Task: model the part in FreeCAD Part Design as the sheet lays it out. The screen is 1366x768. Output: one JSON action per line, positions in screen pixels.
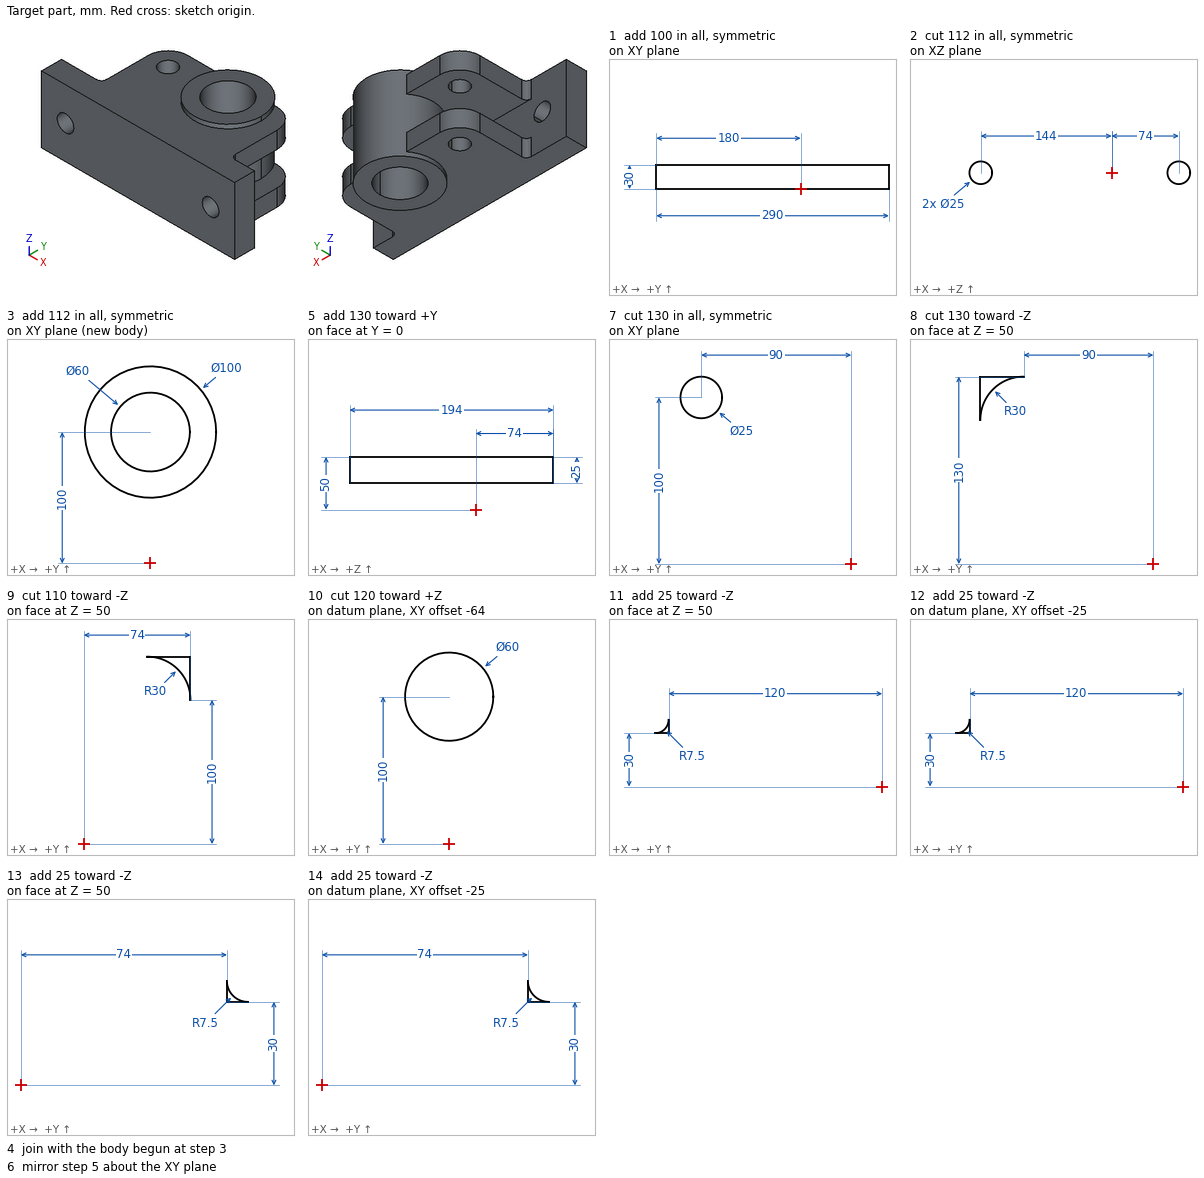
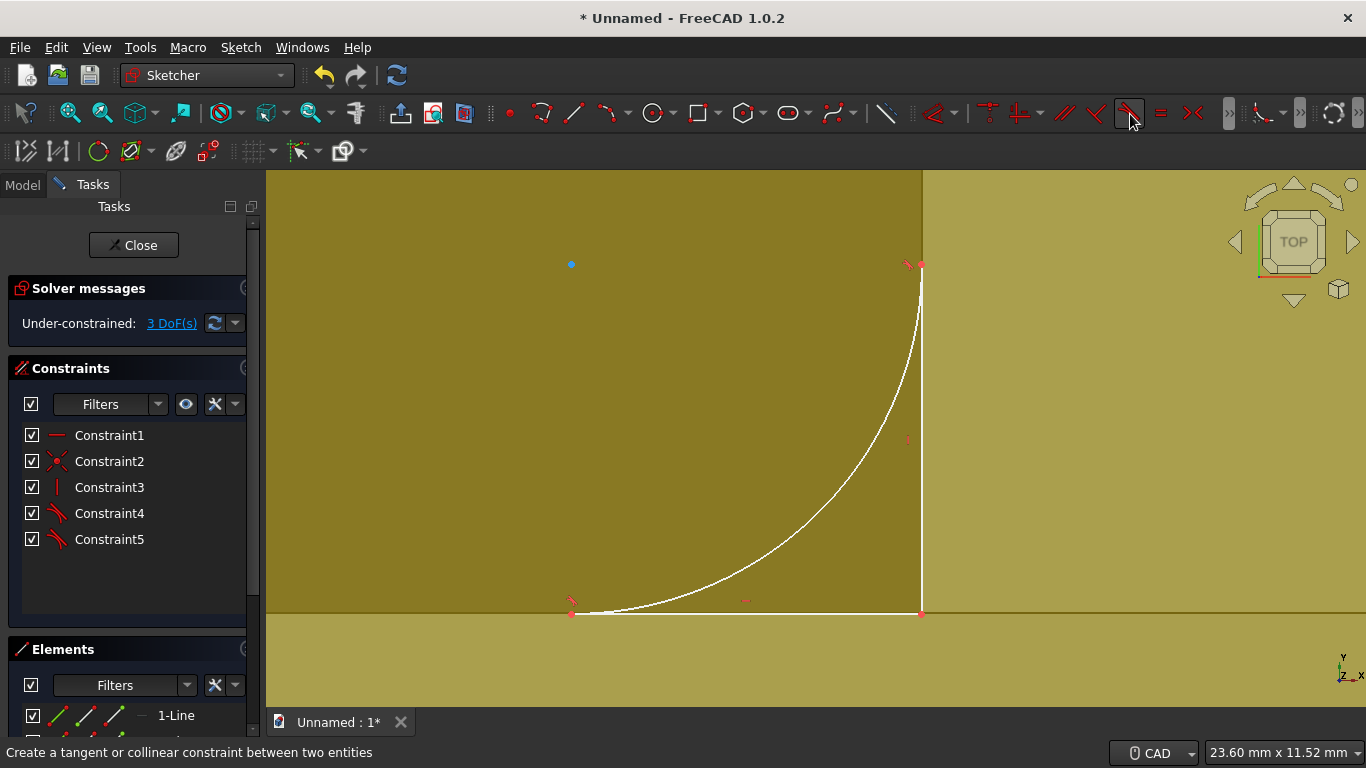
{"action": "left_click", "coordinate": [934, 114]}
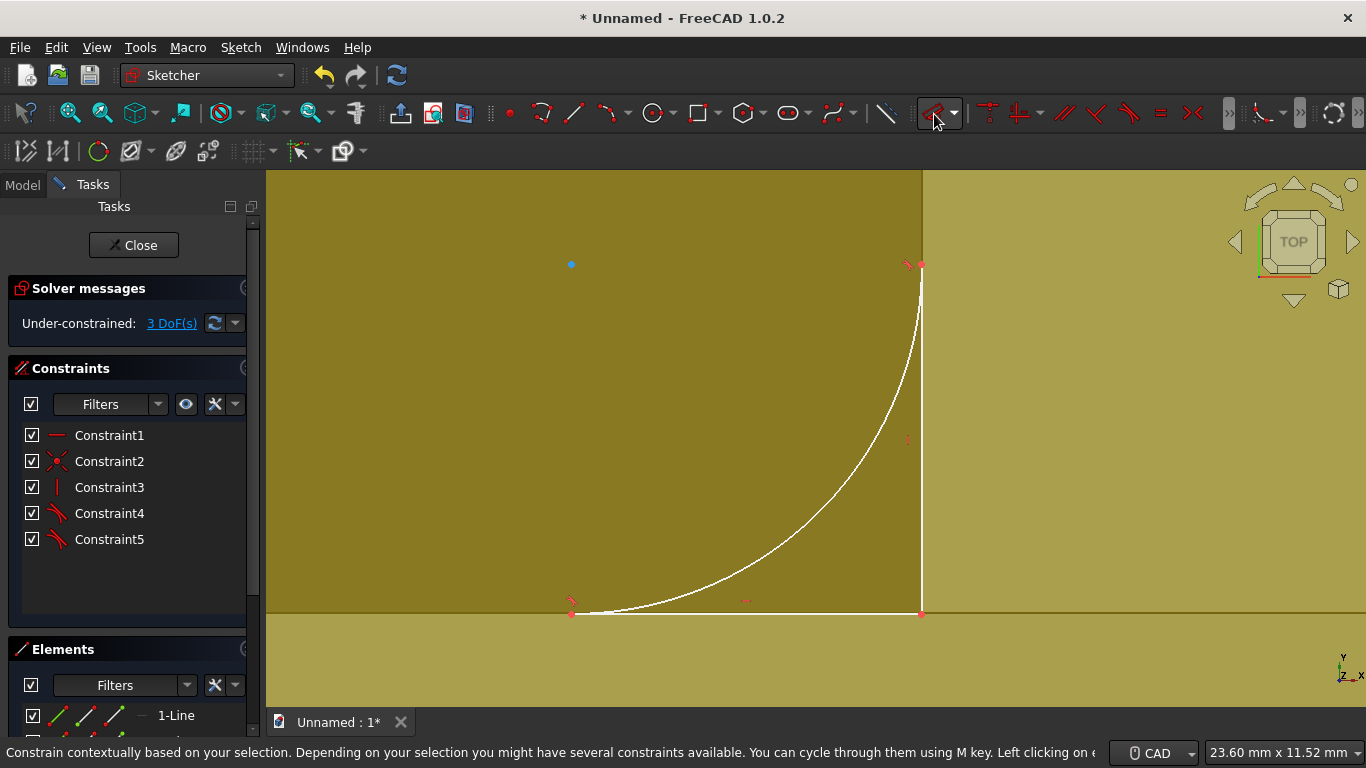
{"action": "left_click", "coordinate": [731, 576]}
{"action": "left_click", "coordinate": [561, 646]}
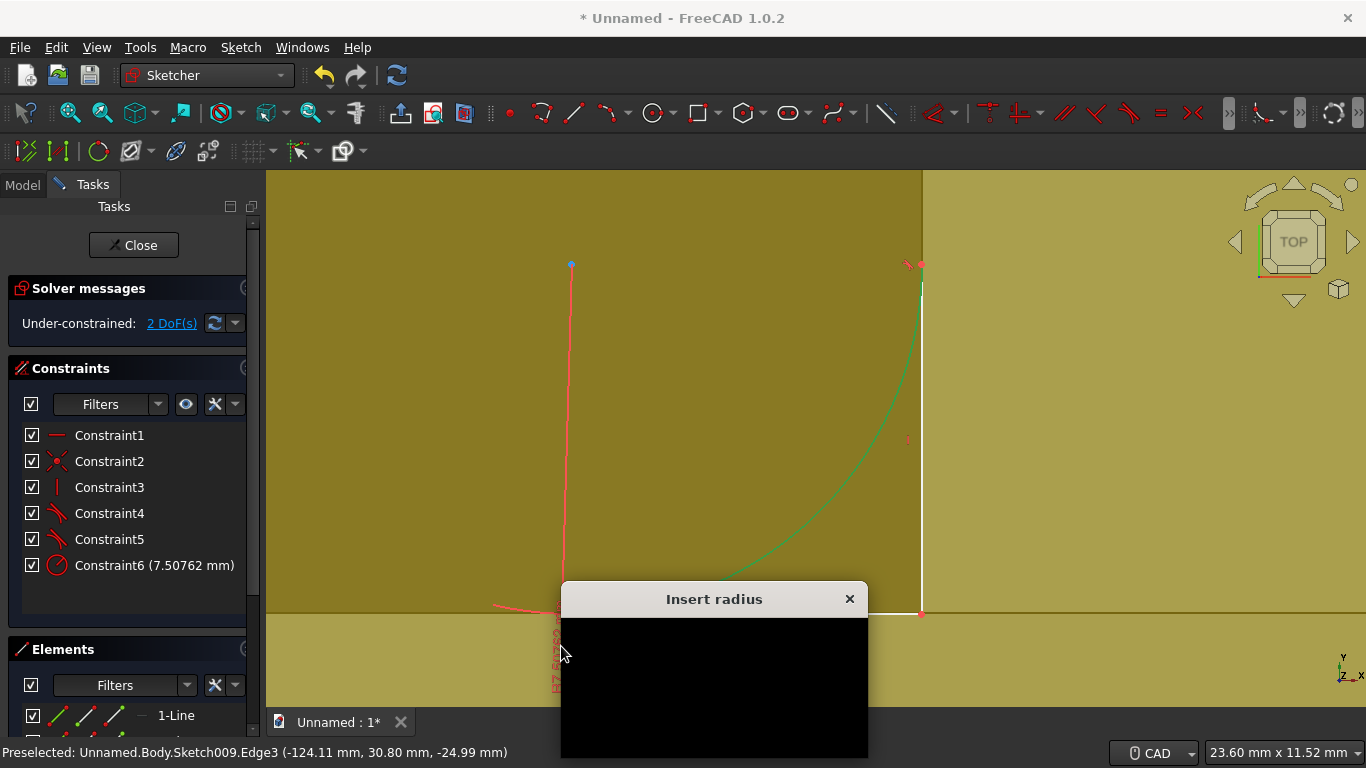
{"action": "type", "text": "7.5"}
{"action": "key", "text": "Return"}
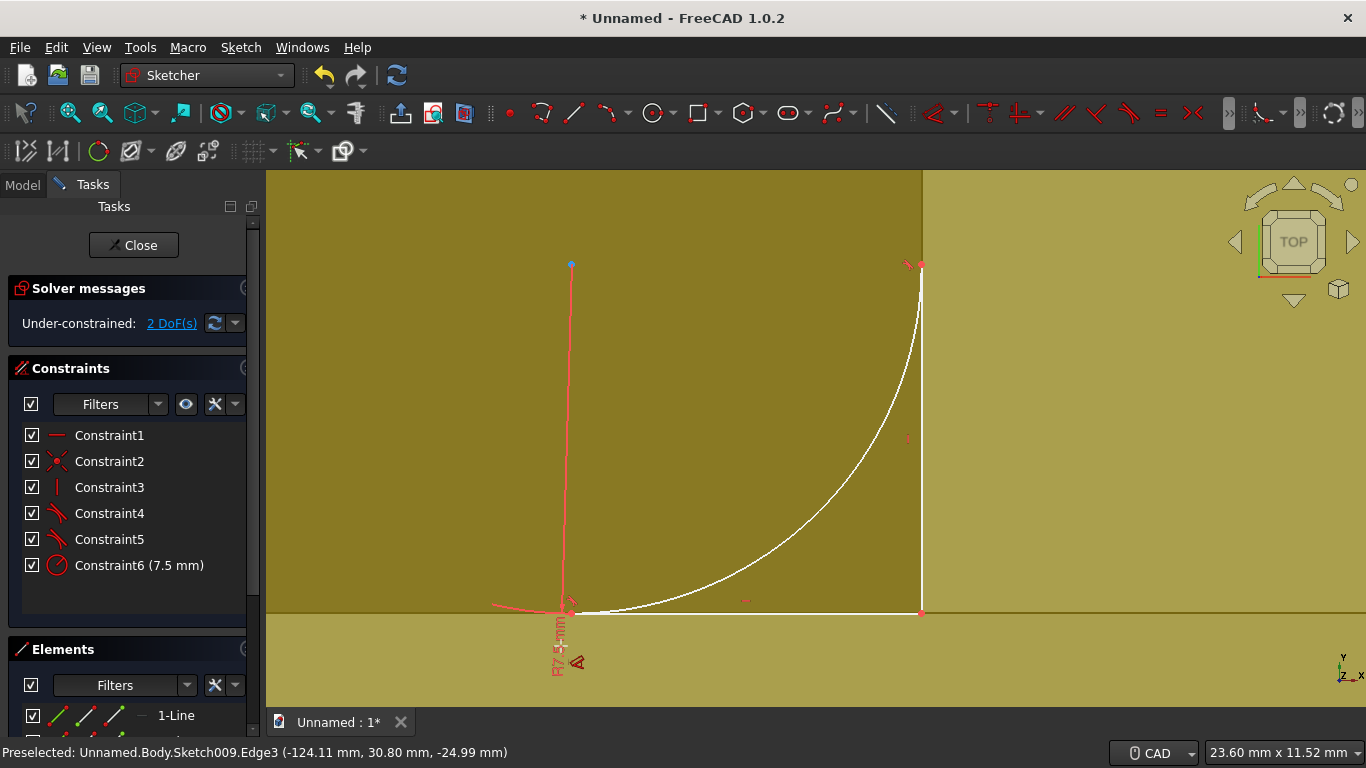
{"action": "left_click", "coordinate": [572, 614]}
{"action": "left_click", "coordinate": [538, 623]}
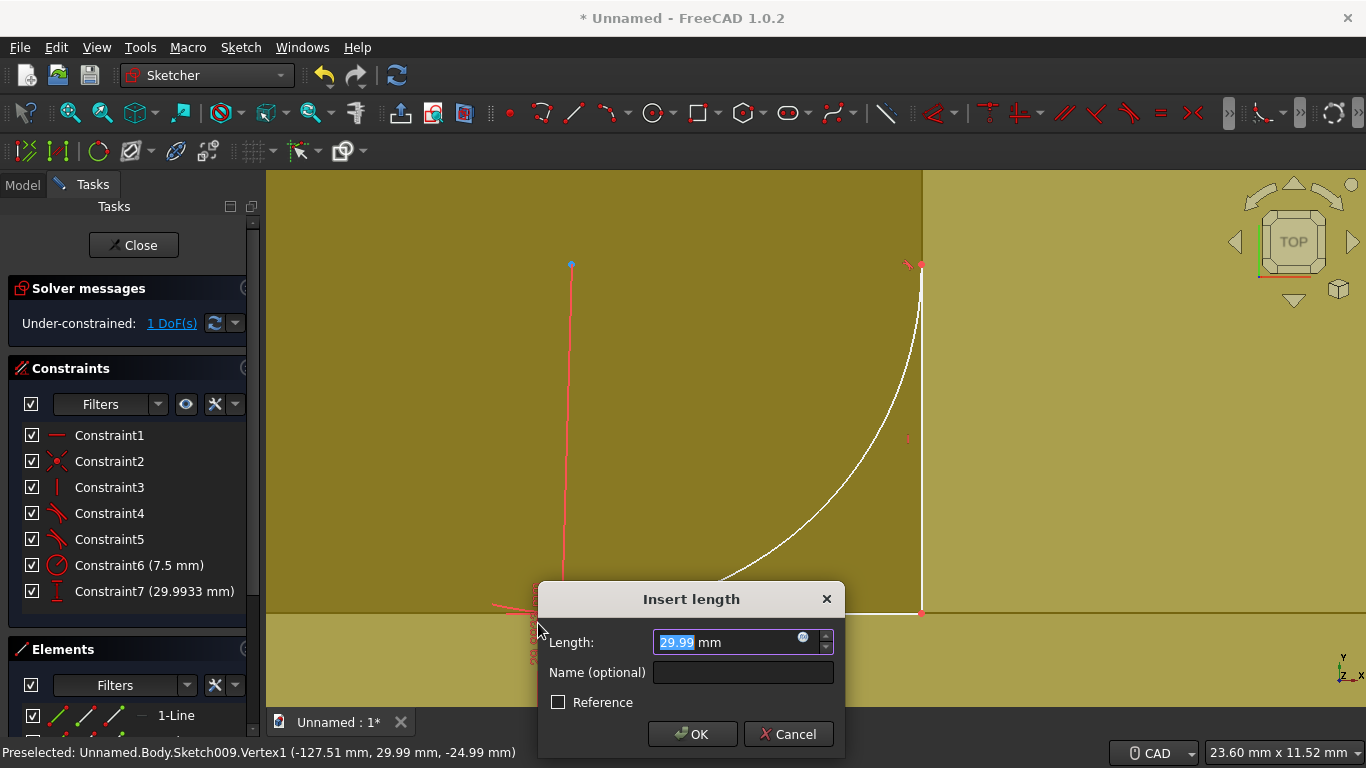
{"action": "type", "text": "30"}
{"action": "key", "text": "Return"}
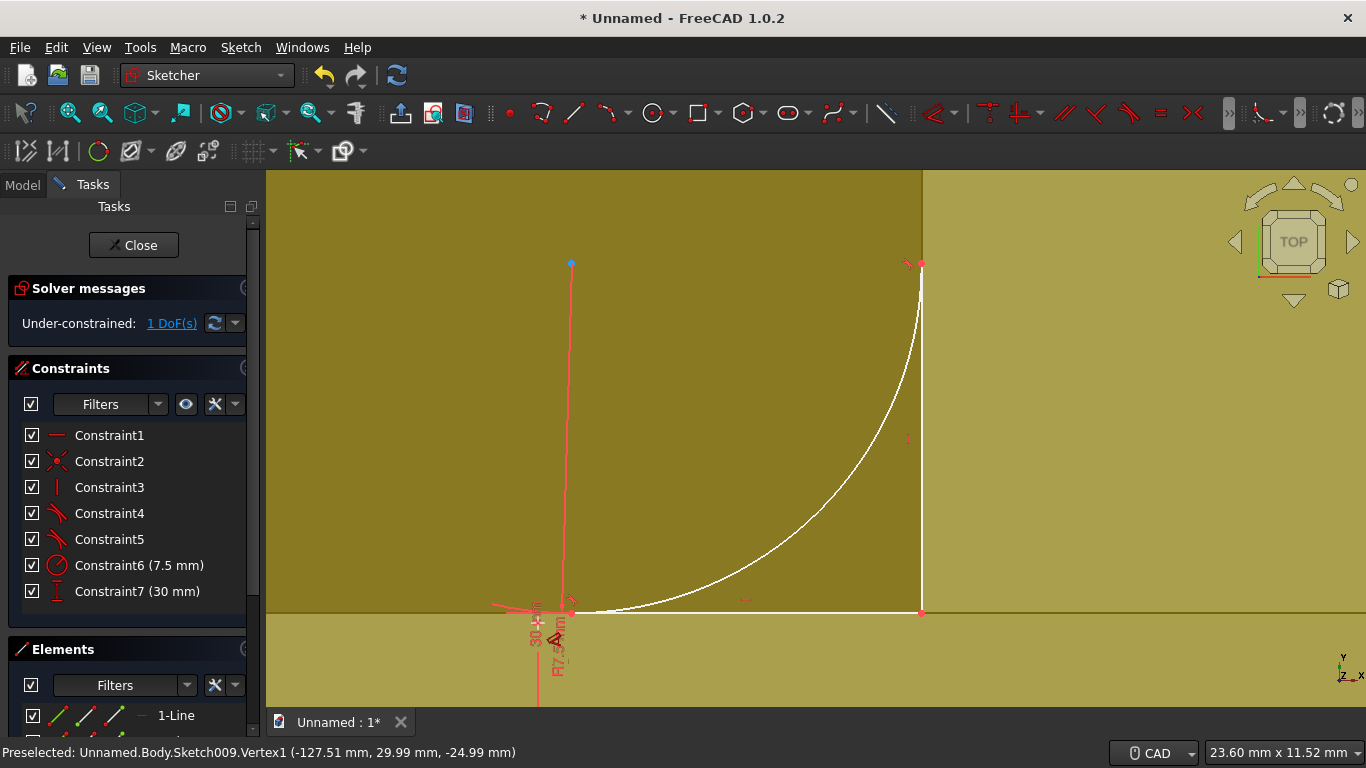
{"action": "left_click", "coordinate": [922, 613]}
{"action": "left_click", "coordinate": [1061, 579]}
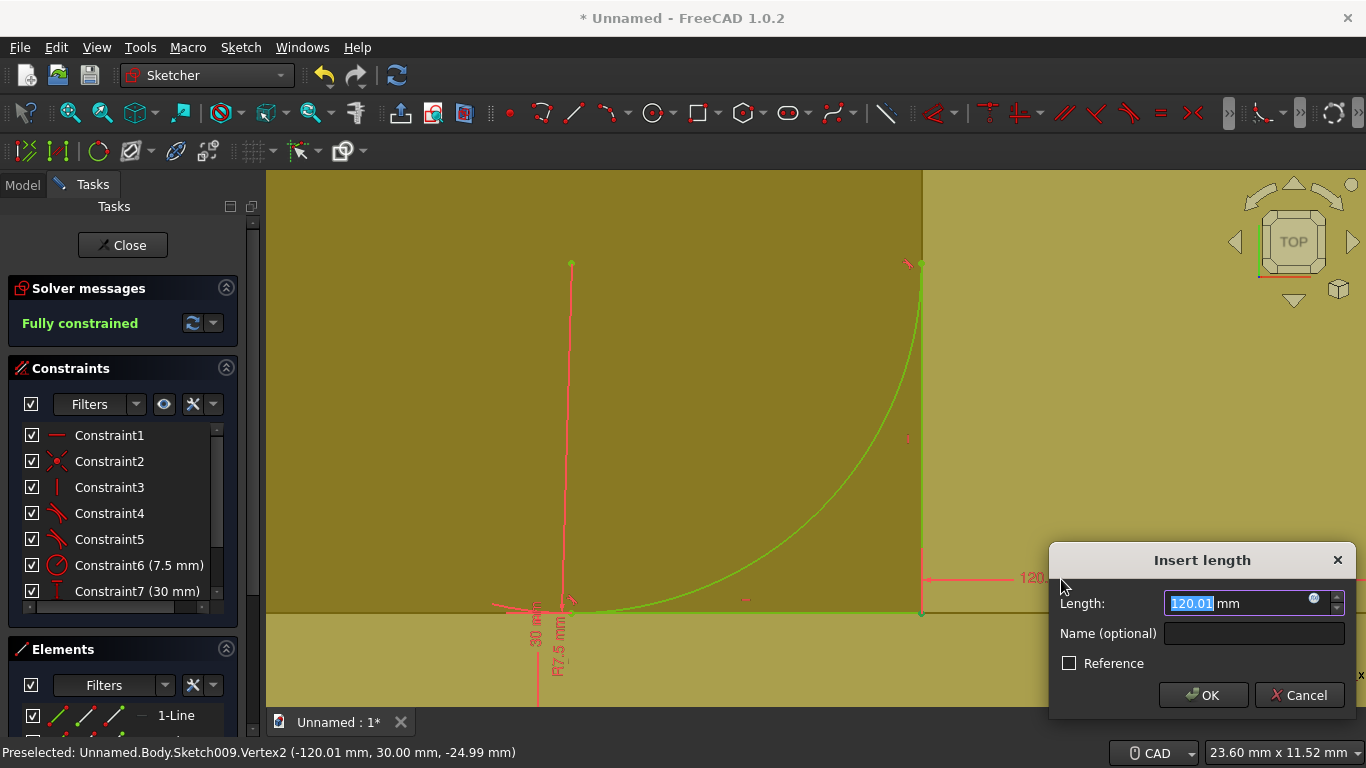
{"action": "type", "text": "120"}
{"action": "key", "text": "Return"}
{"action": "key", "text": "Escape"}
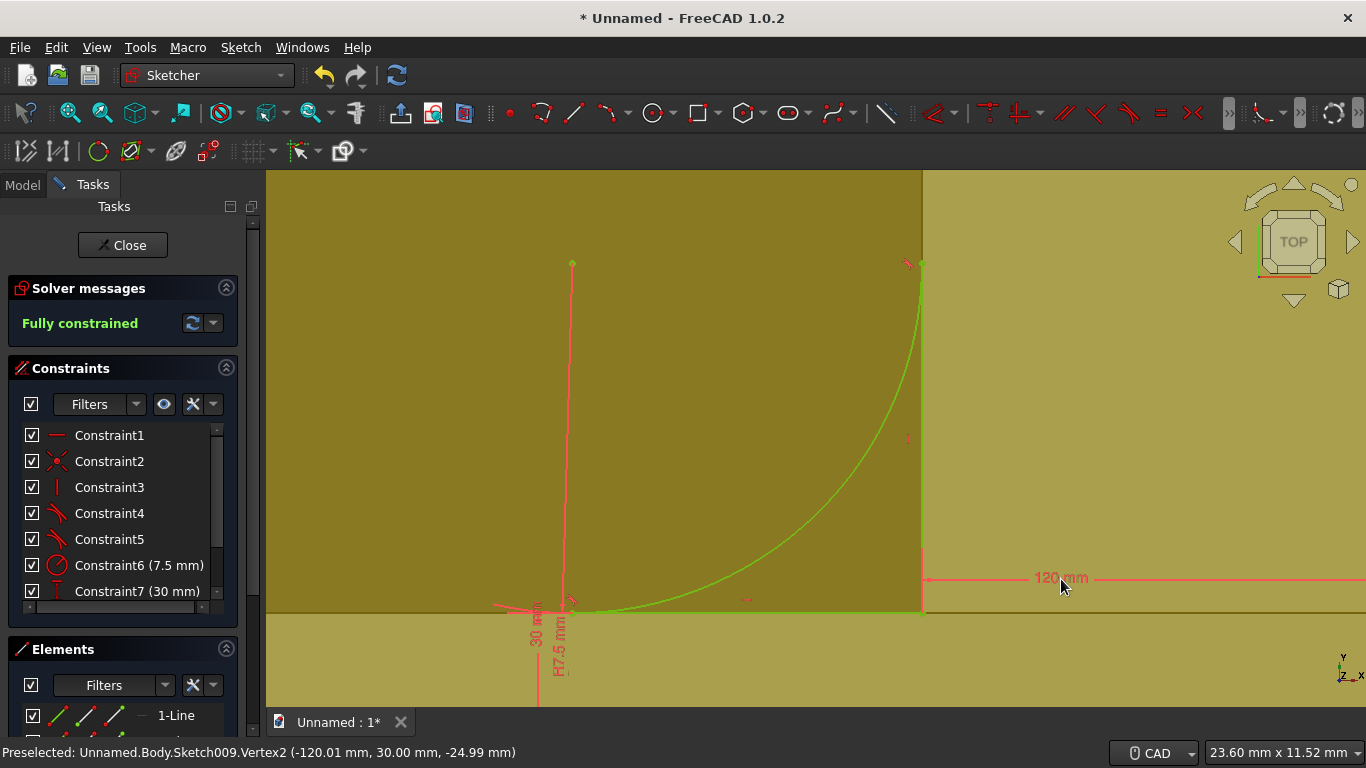
{"action": "left_click", "coordinate": [123, 245]}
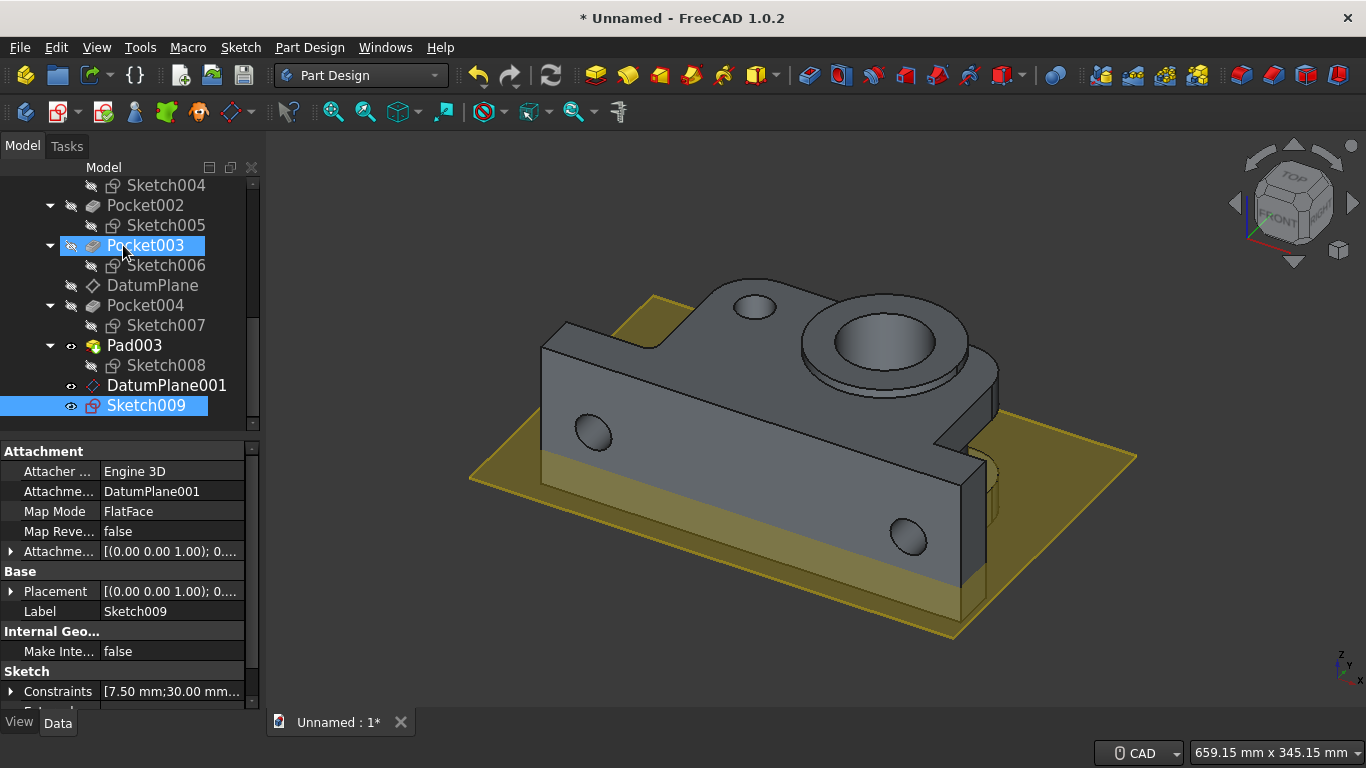
{"action": "left_click", "coordinate": [596, 76]}